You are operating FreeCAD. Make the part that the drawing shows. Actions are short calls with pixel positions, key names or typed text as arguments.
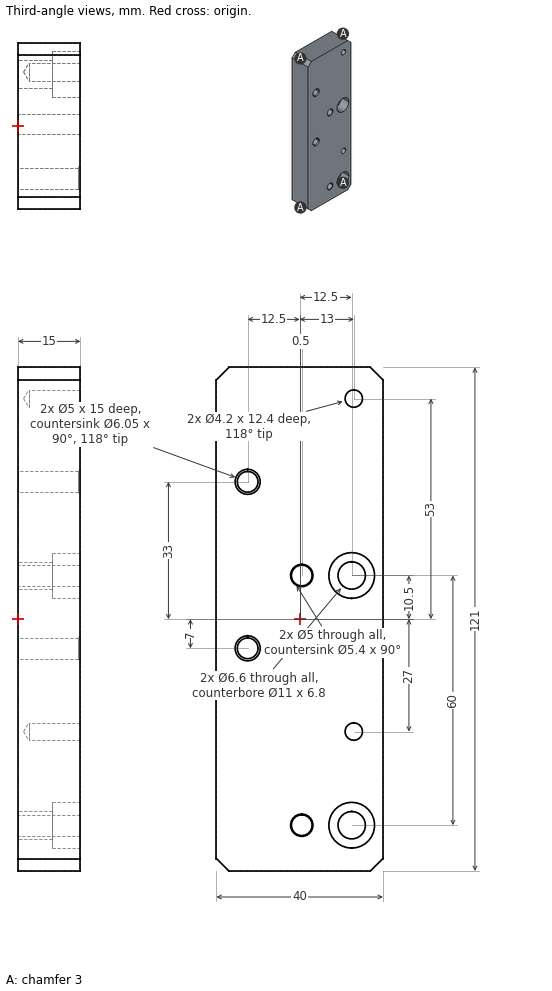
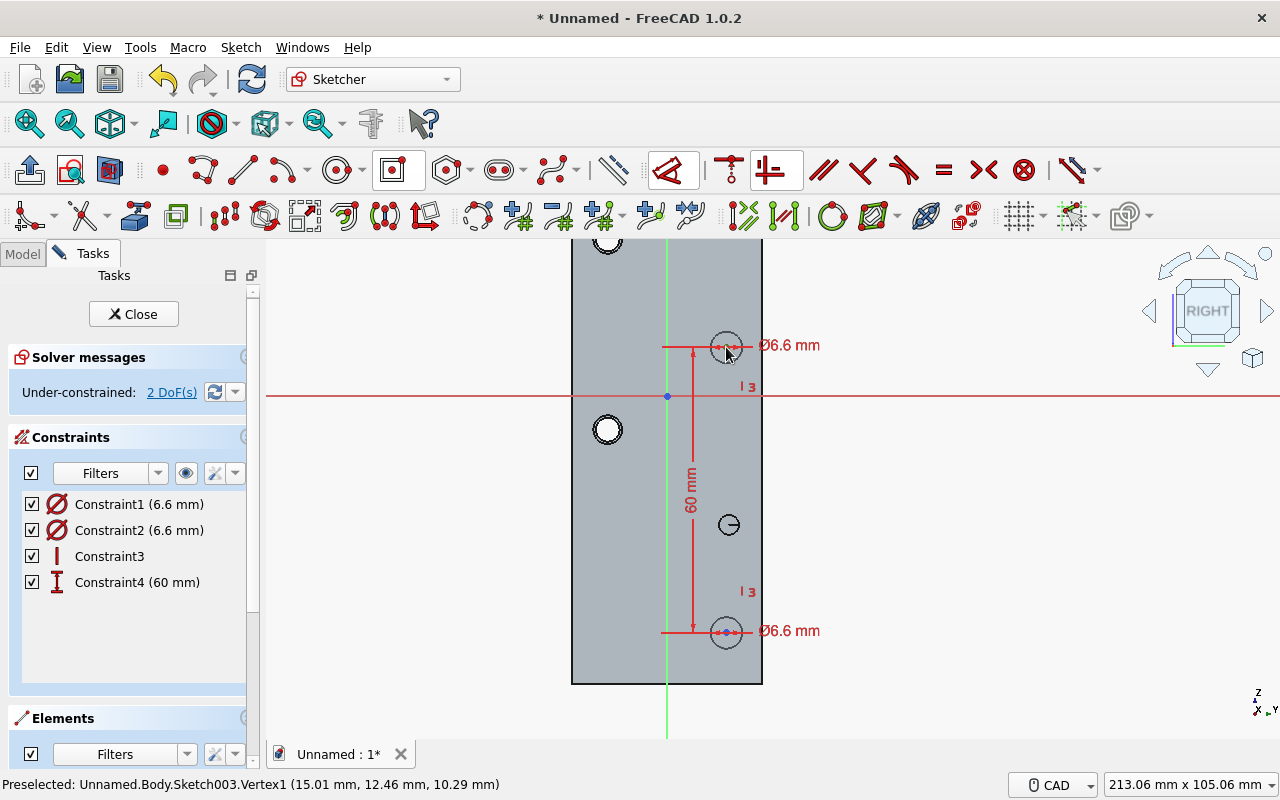
key(l)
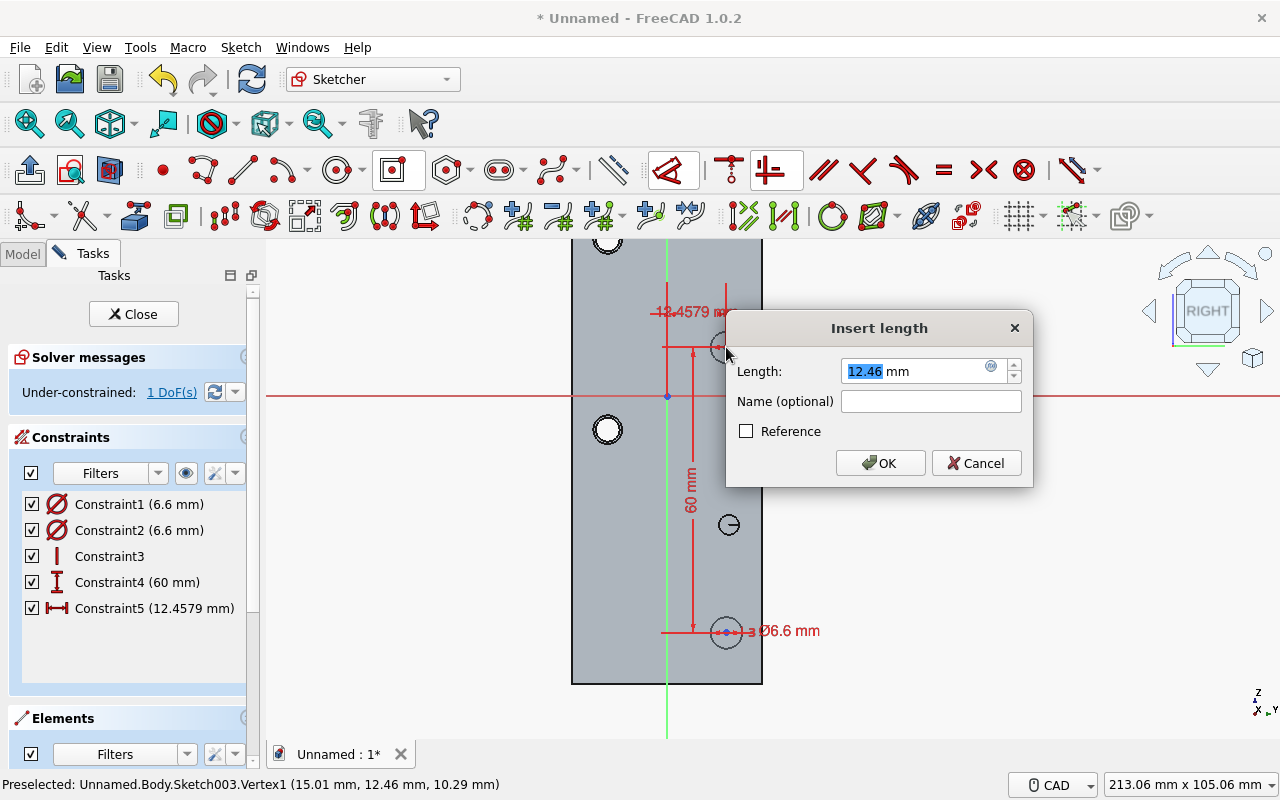
text(12.5)
key(Return)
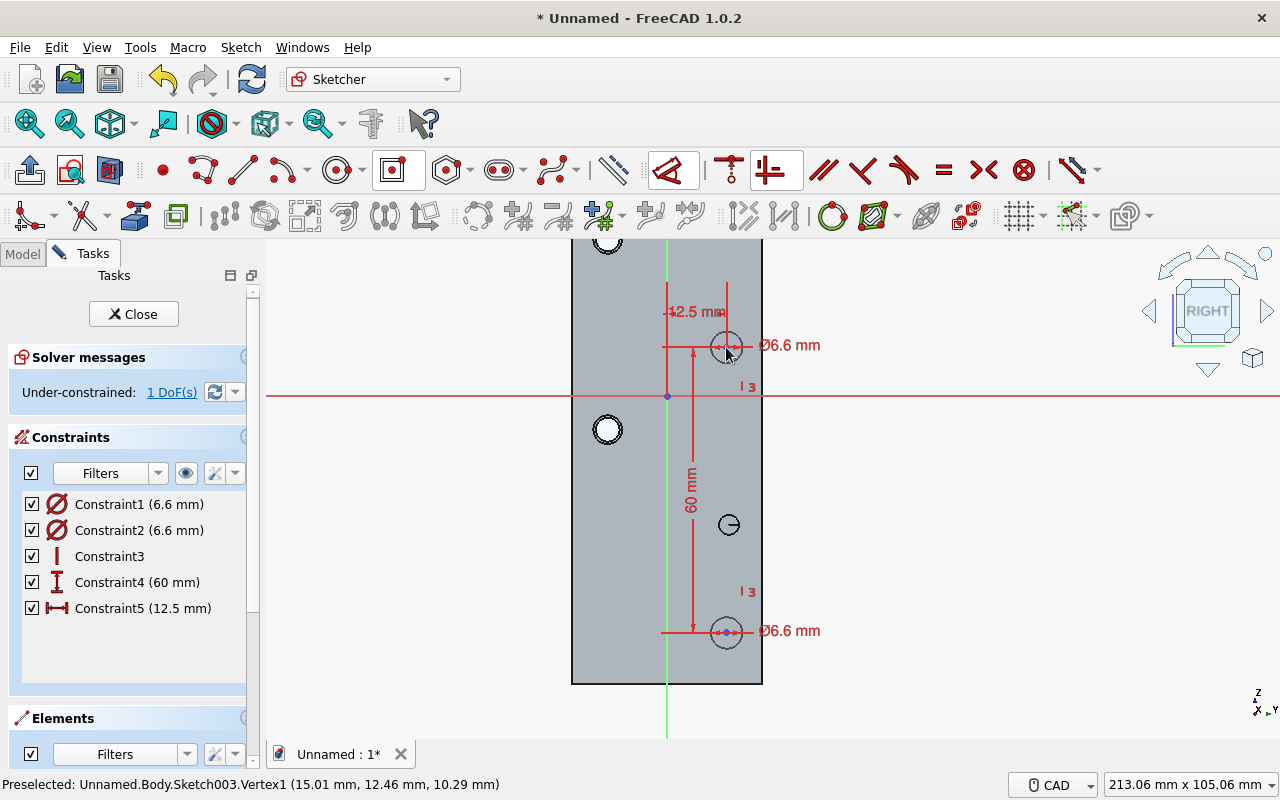
click(727, 347)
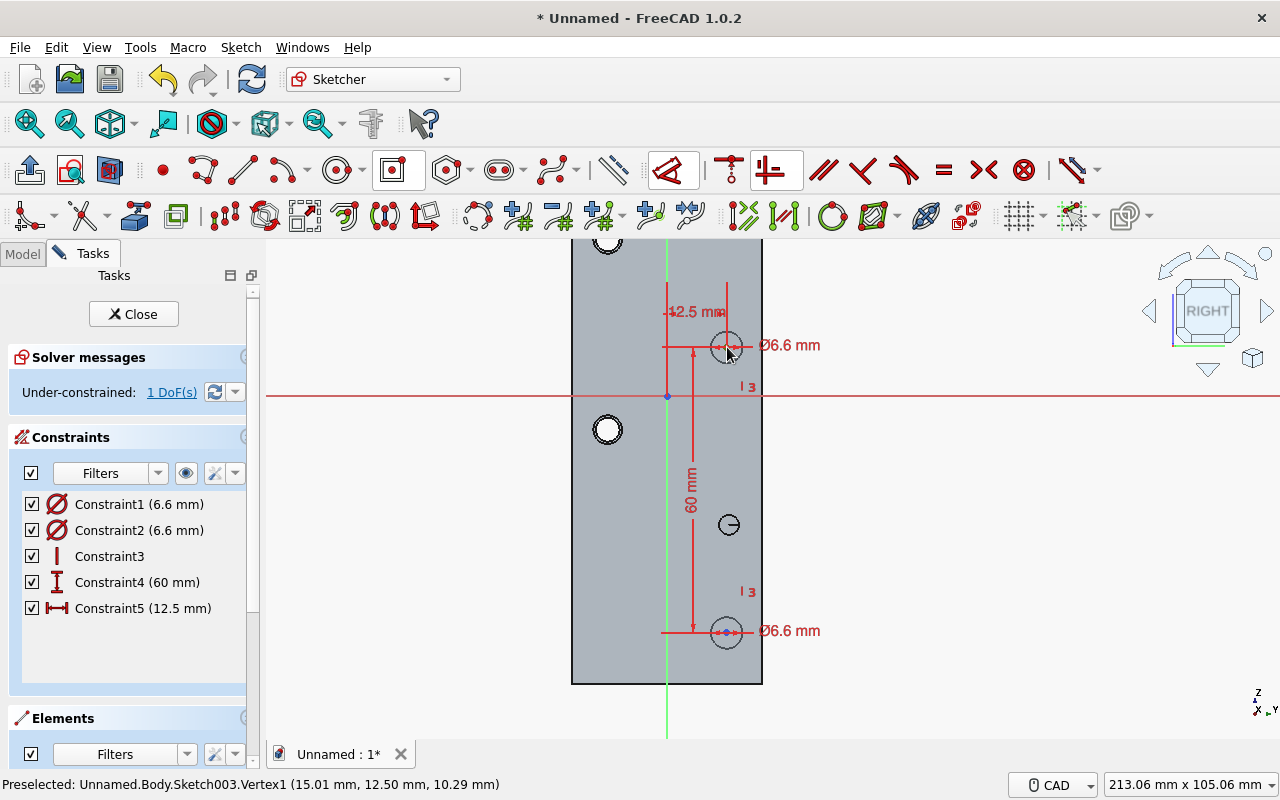
click(694, 170)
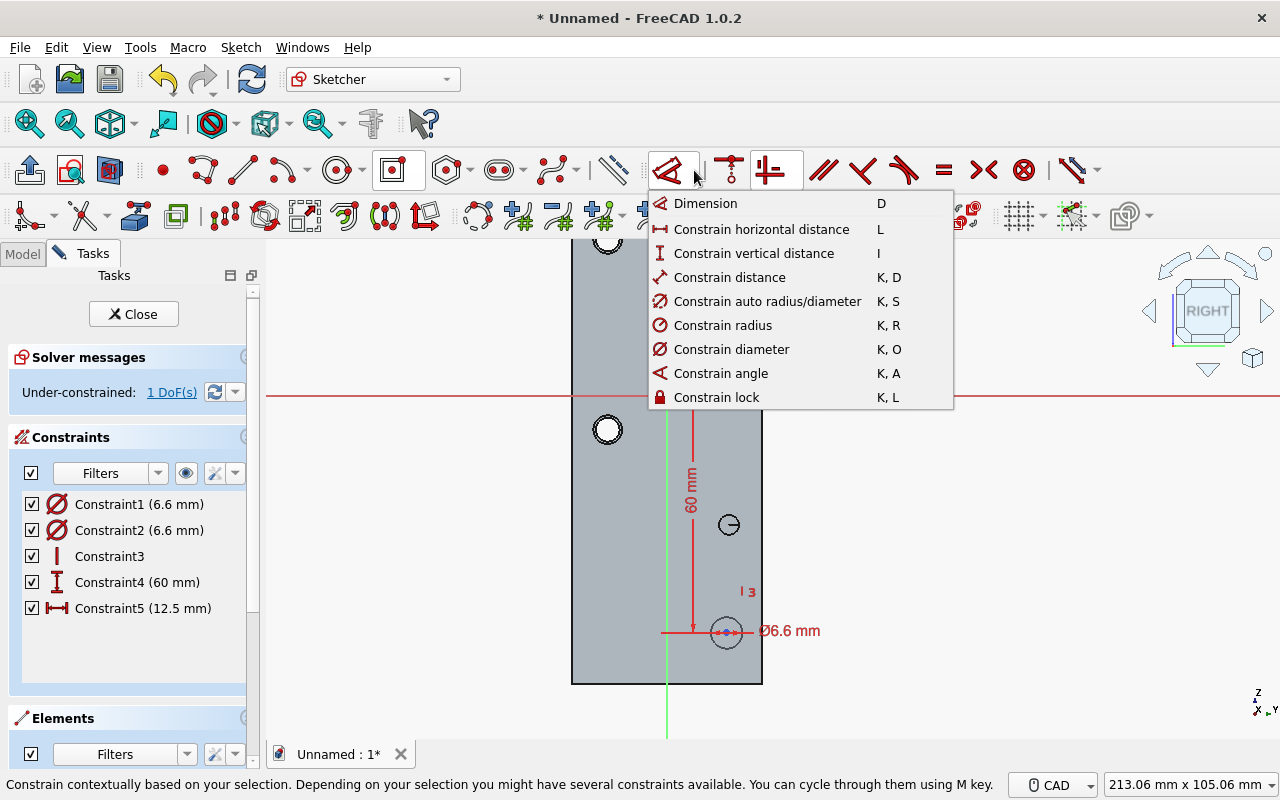
click(801, 253)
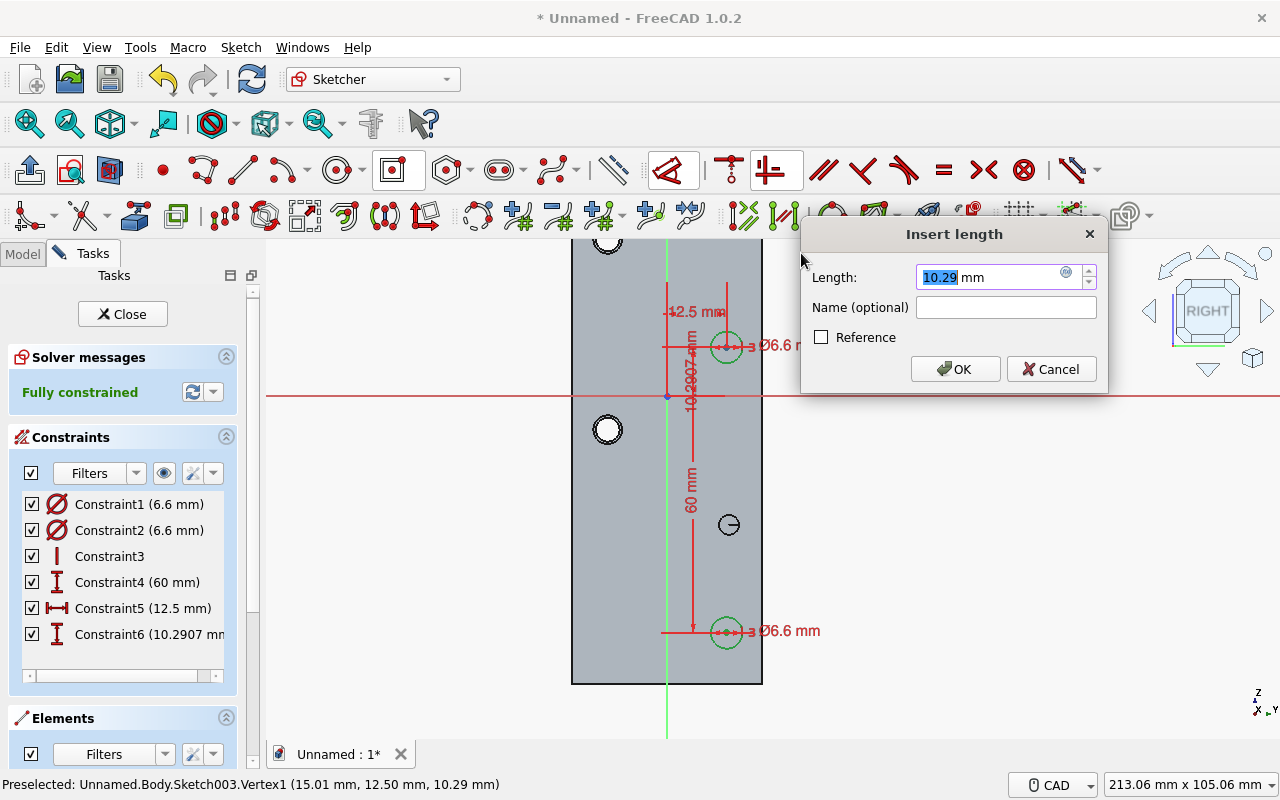
text(10.5)
key(Return)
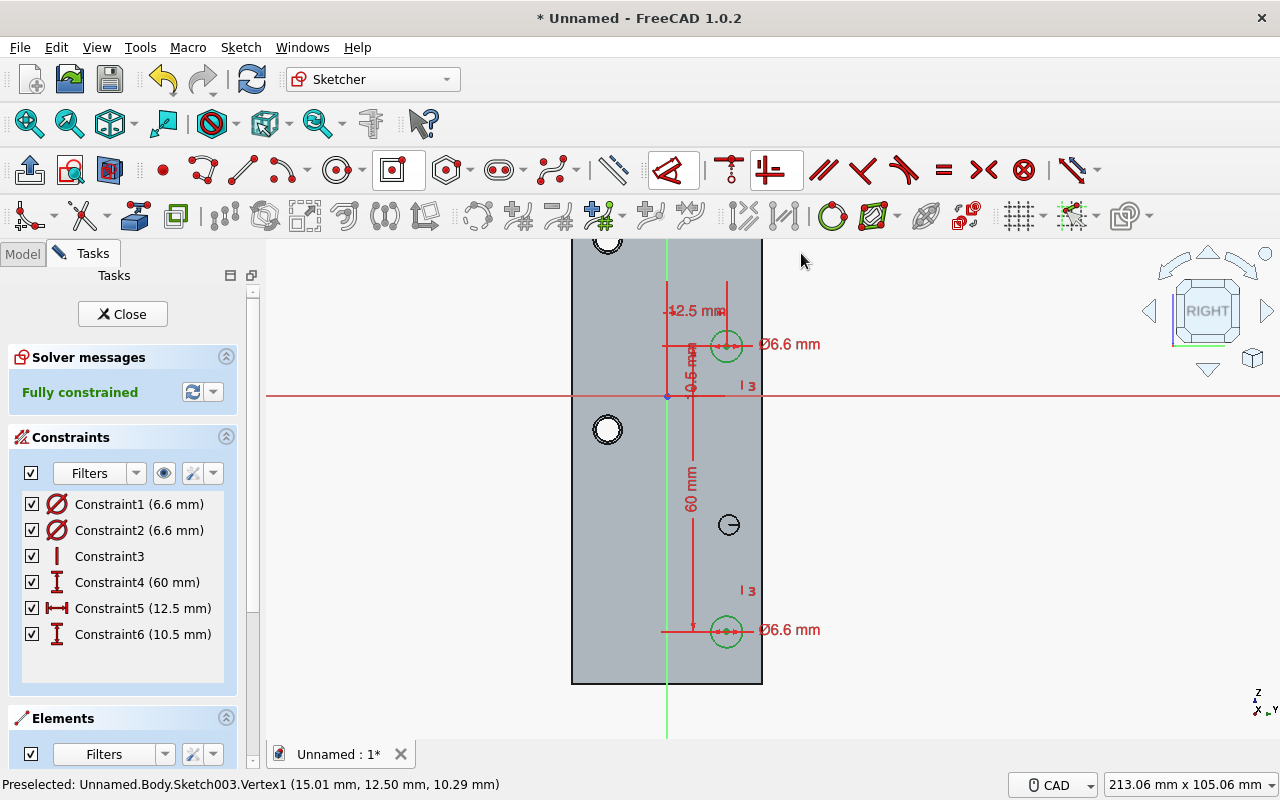
click(123, 314)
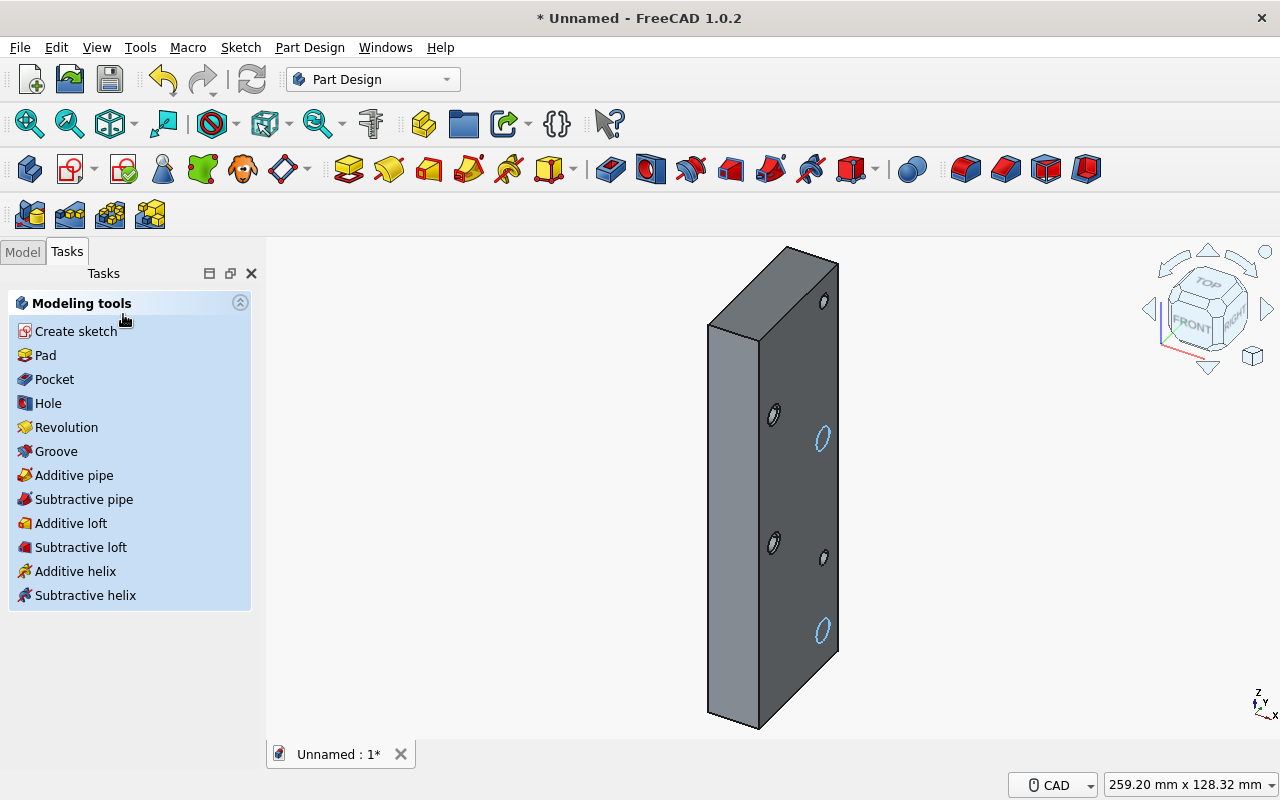
click(652, 170)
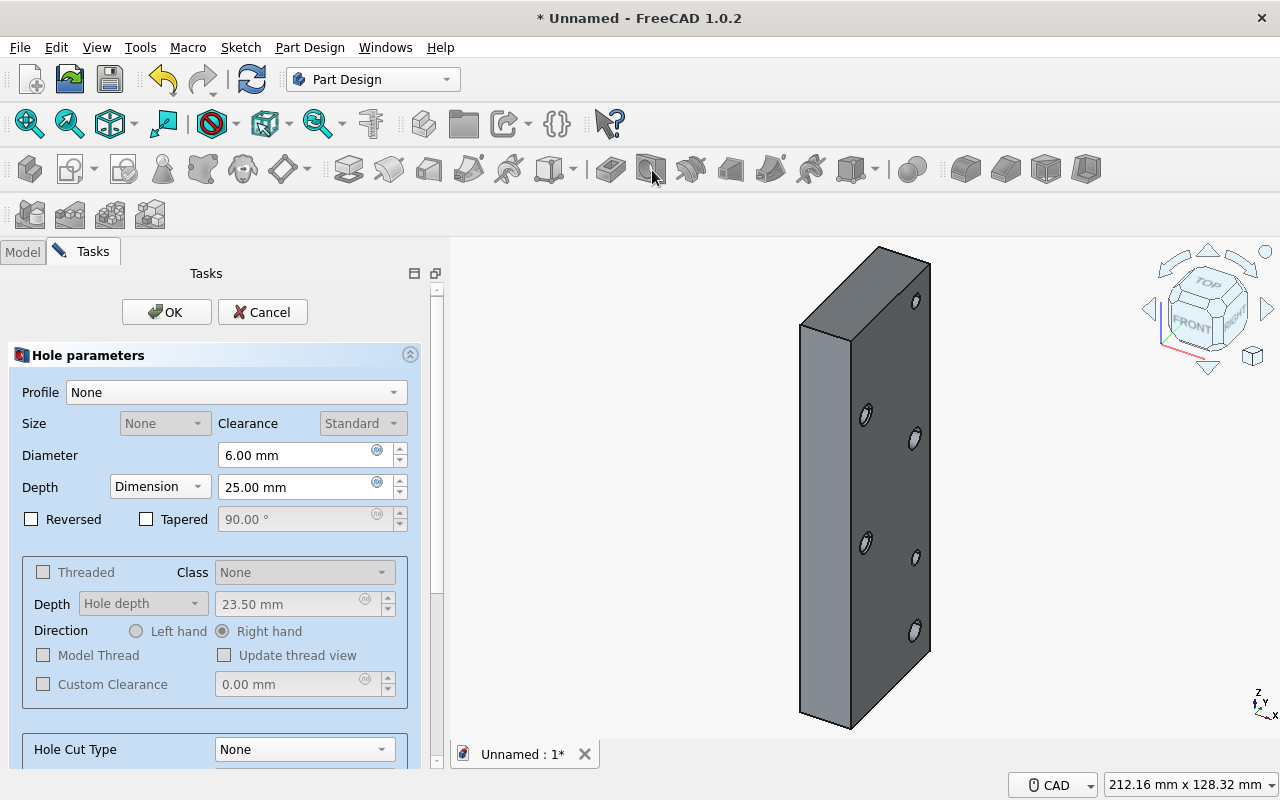
triple_click(305, 455)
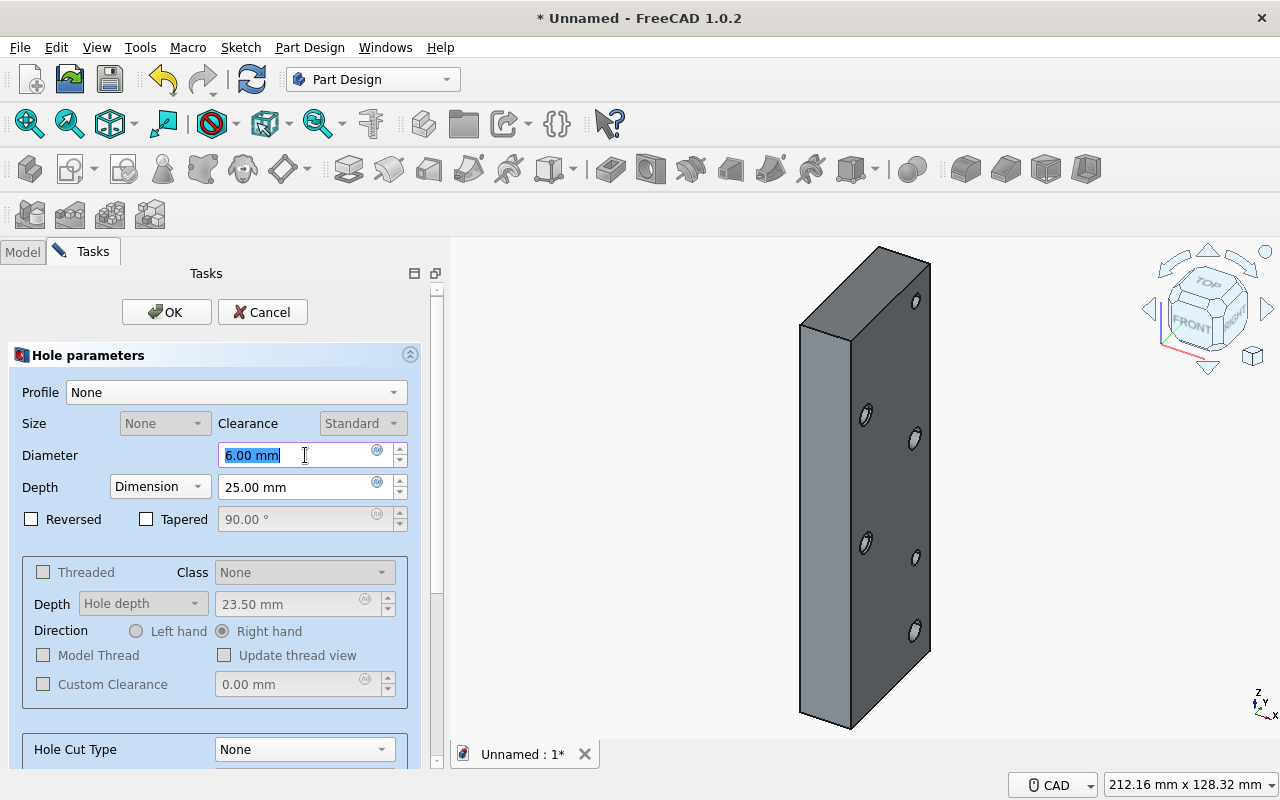
text(6.6)
key(Tab)